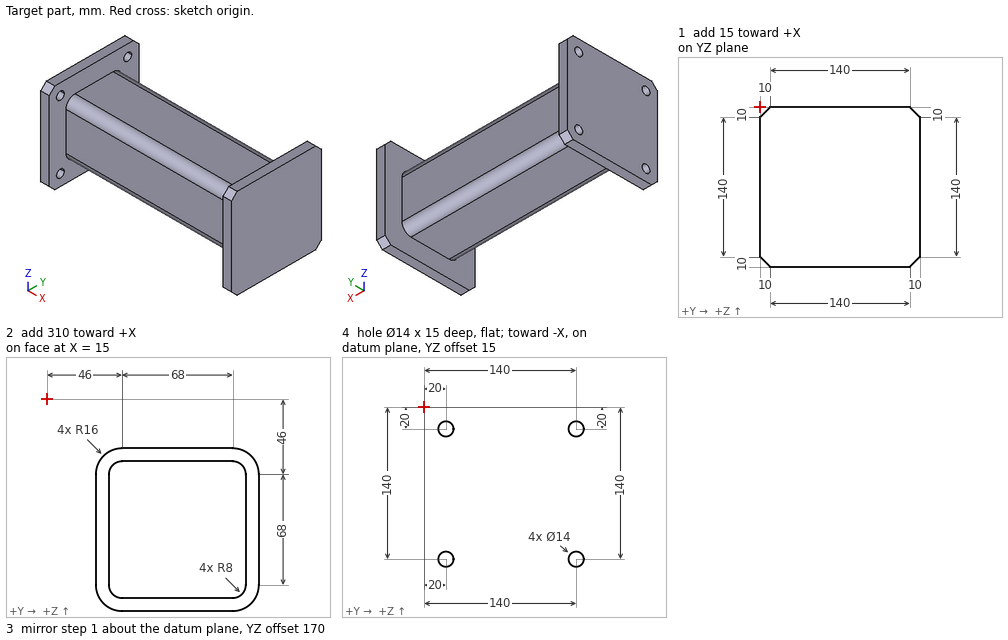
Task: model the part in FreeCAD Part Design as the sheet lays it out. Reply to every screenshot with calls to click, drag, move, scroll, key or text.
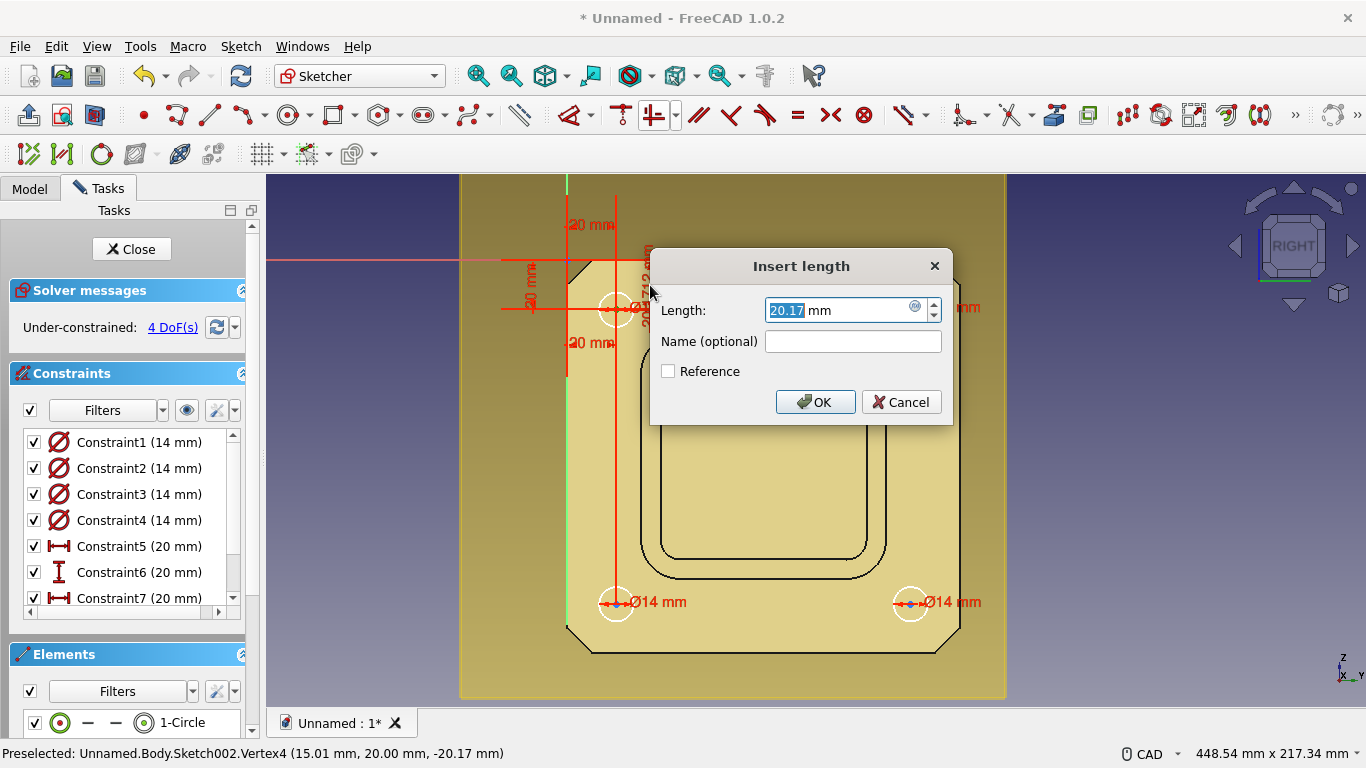
text(20)
key(Return)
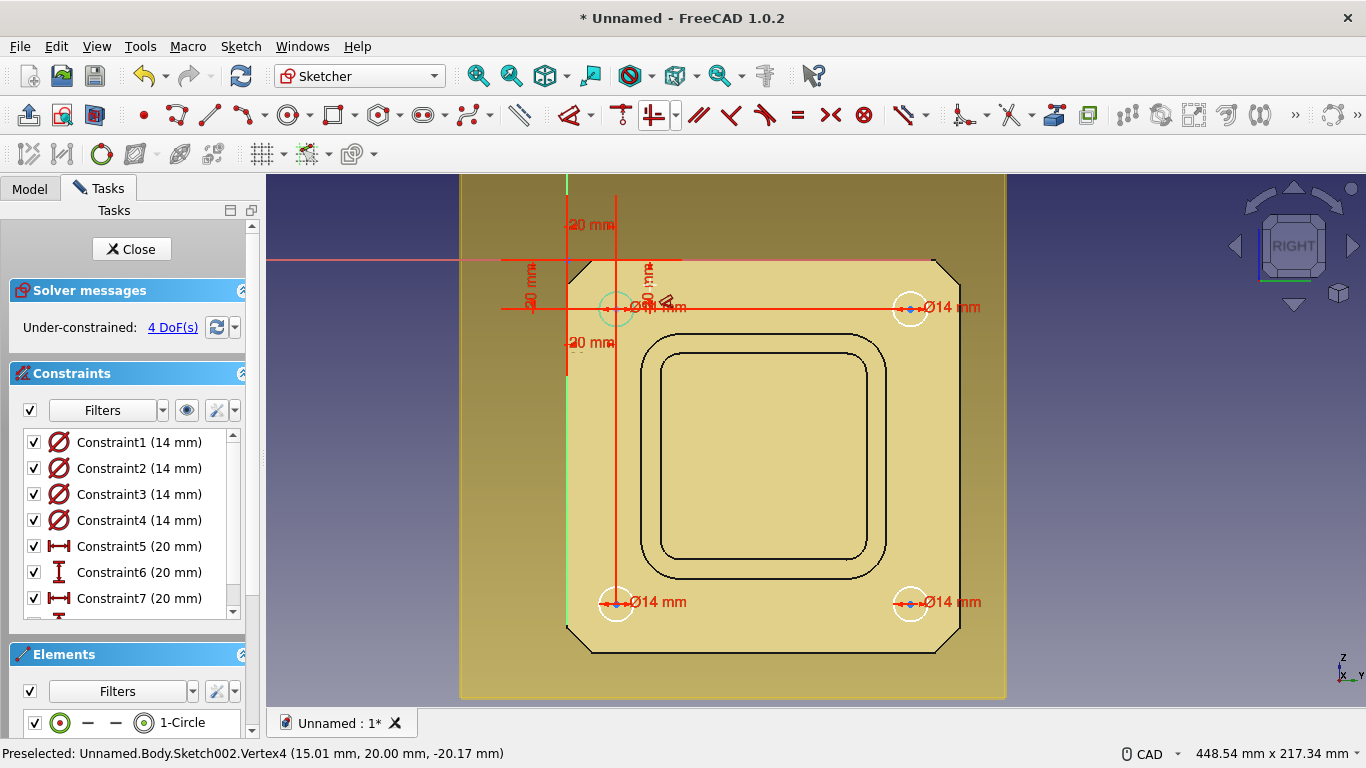
click(911, 604)
click(739, 226)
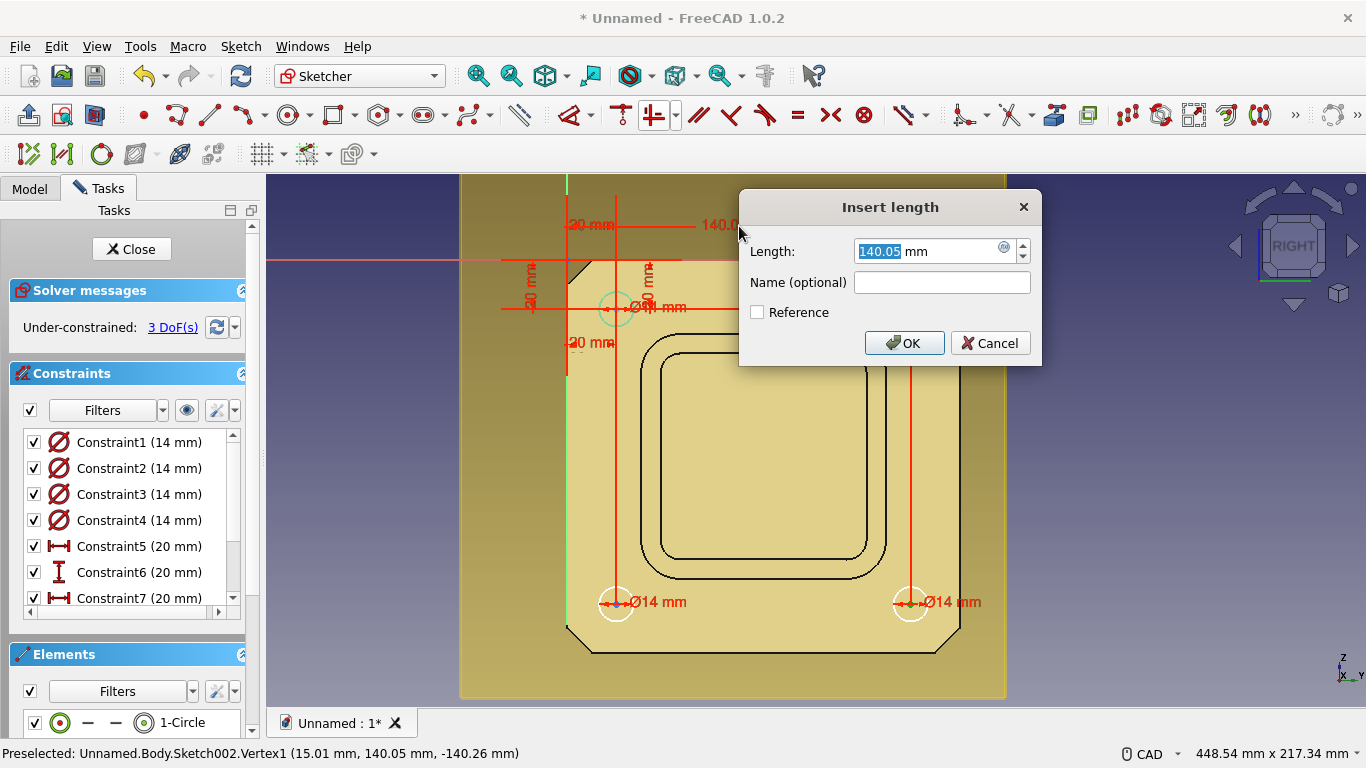
text(140)
key(Return)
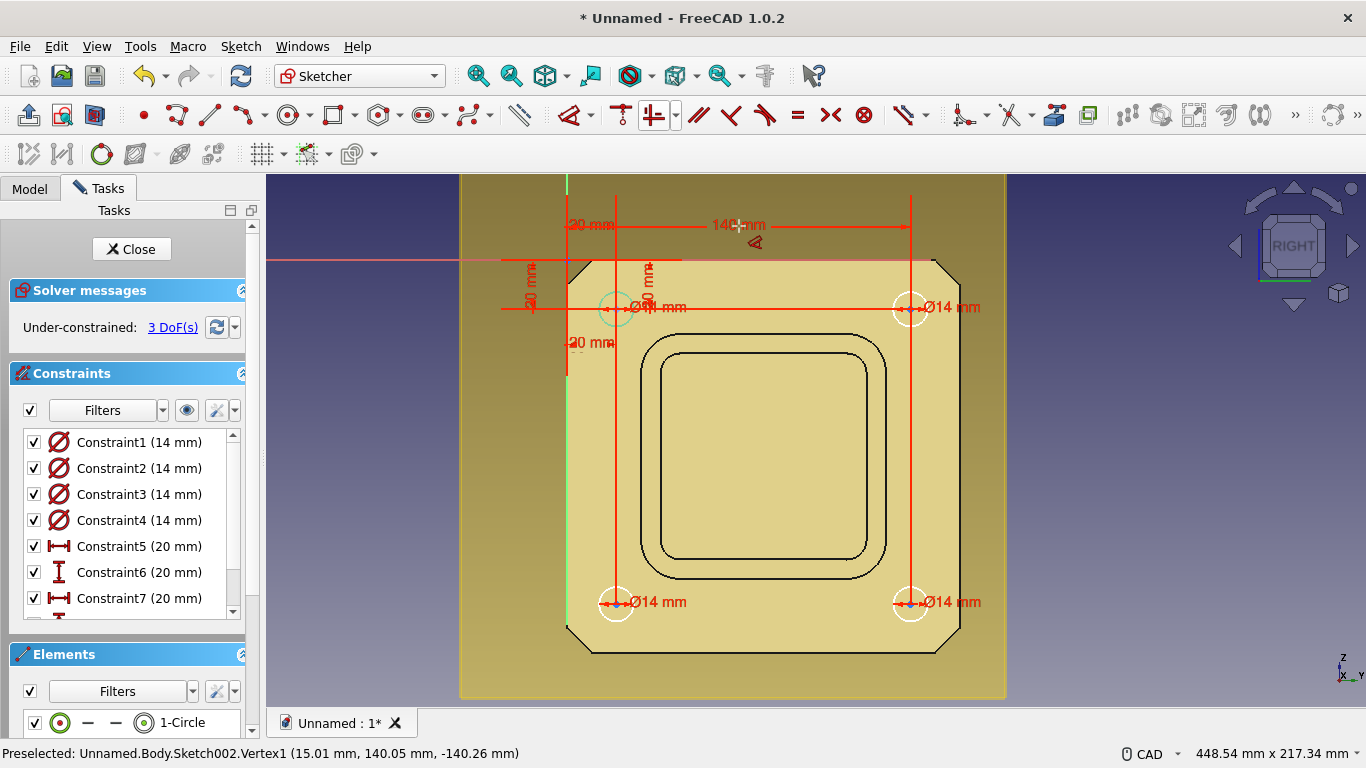
click(911, 604)
click(533, 432)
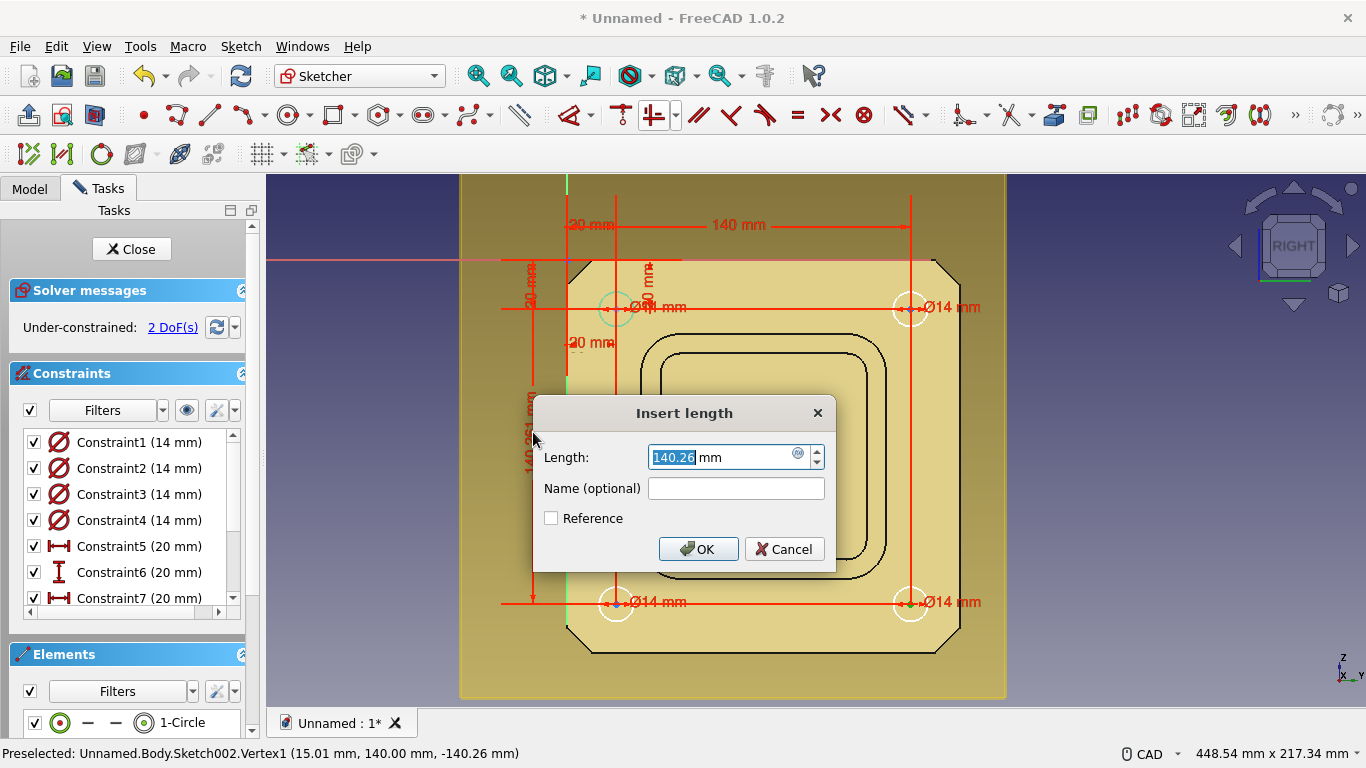
text(140)
key(Return)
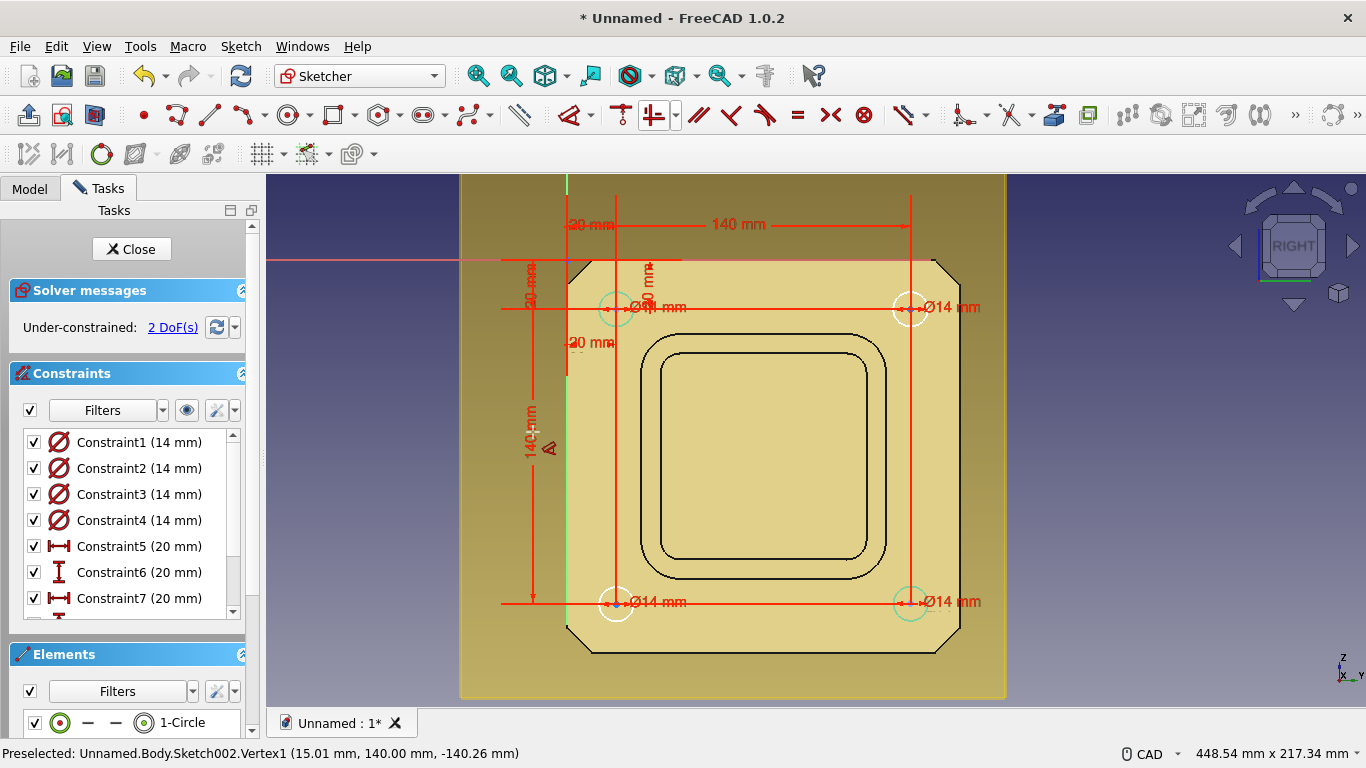
click(616, 604)
click(533, 511)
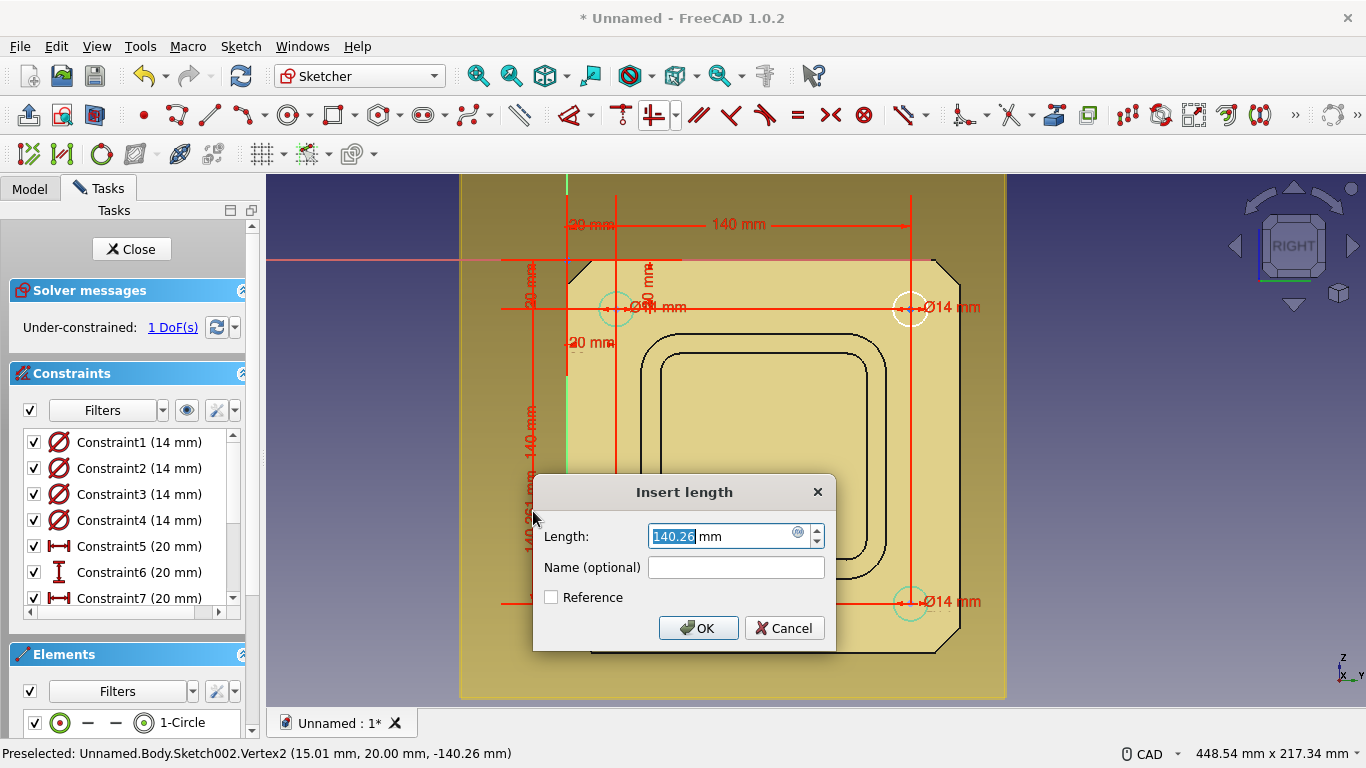
text(140)
key(Return)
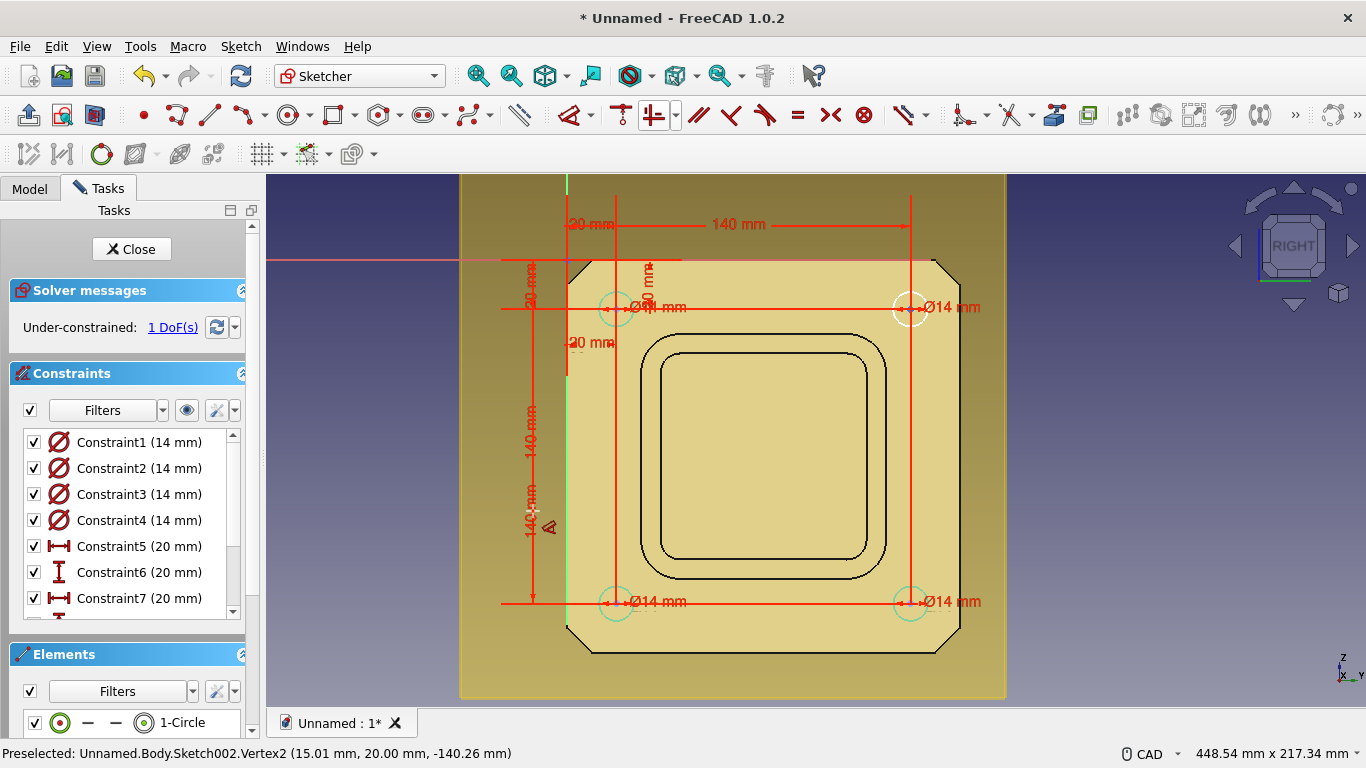
click(911, 309)
click(818, 226)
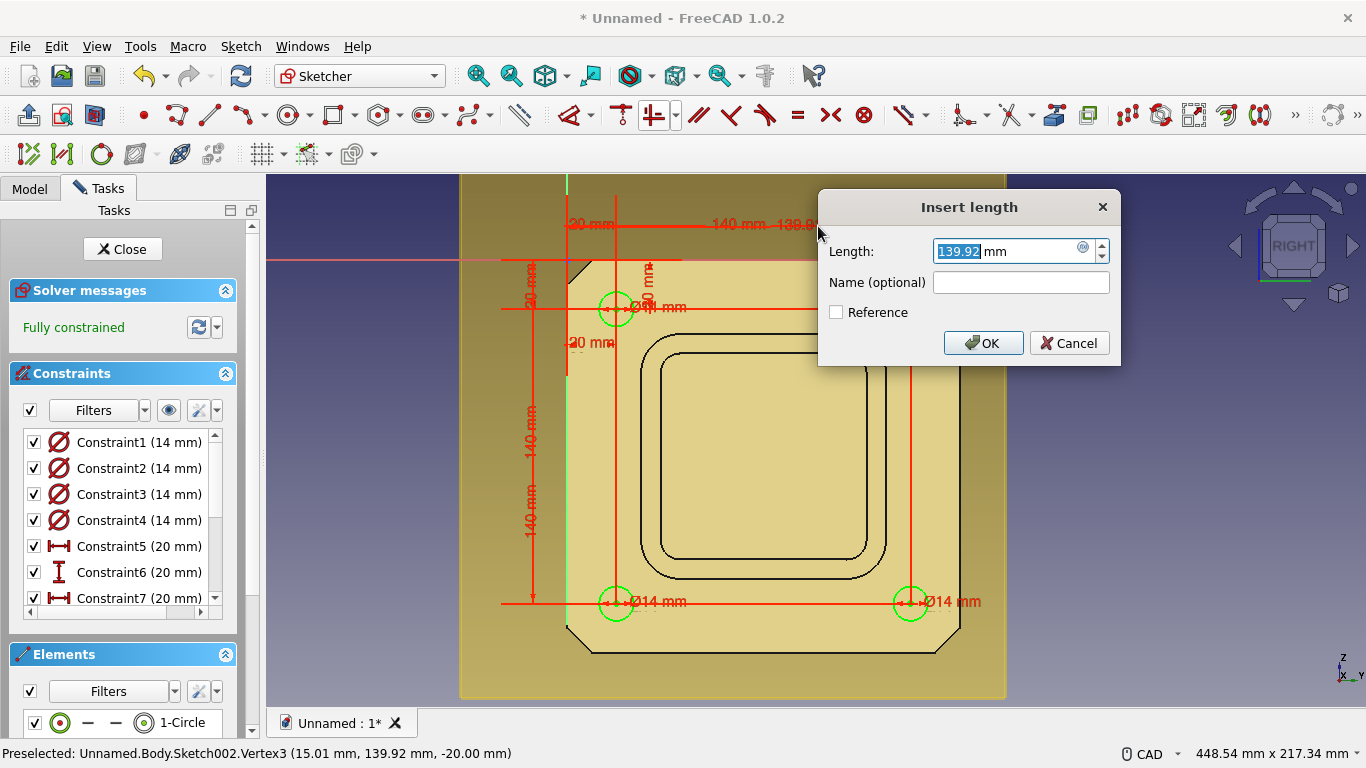
text(140)
key(Return)
key(Escape)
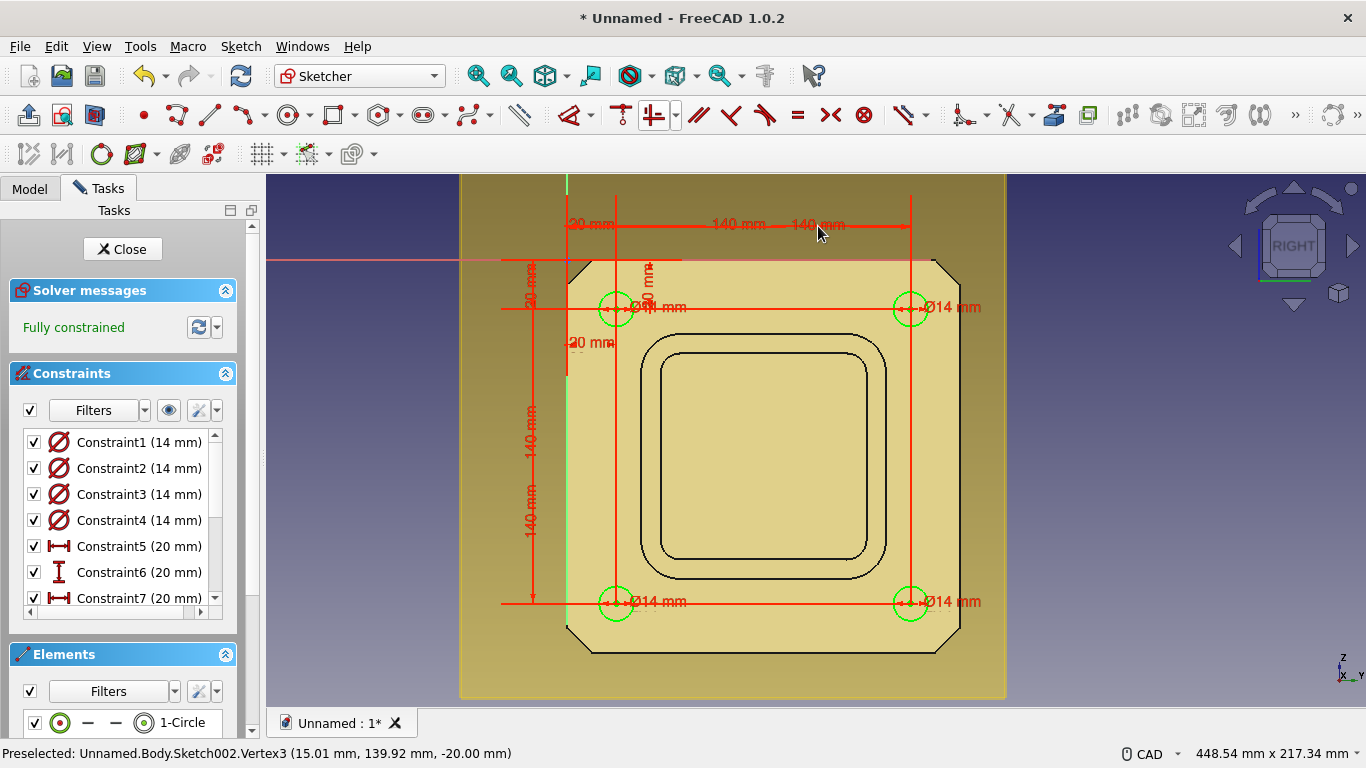
click(123, 249)